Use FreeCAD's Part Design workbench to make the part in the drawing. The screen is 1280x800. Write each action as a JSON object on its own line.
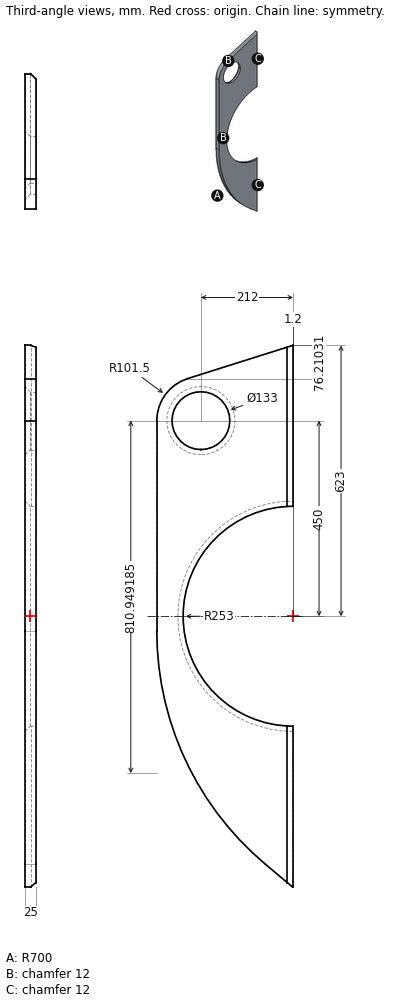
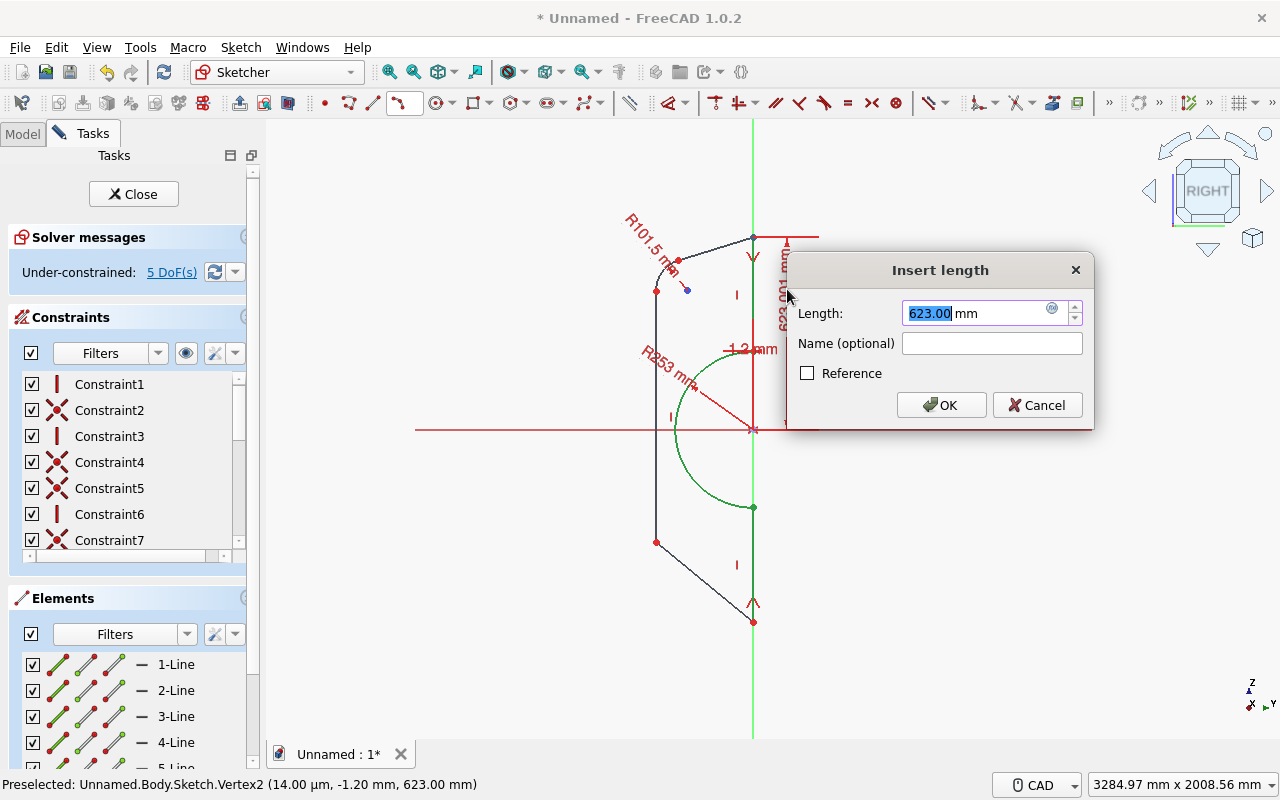
{"action": "type", "text": "623"}
{"action": "key", "text": "Return"}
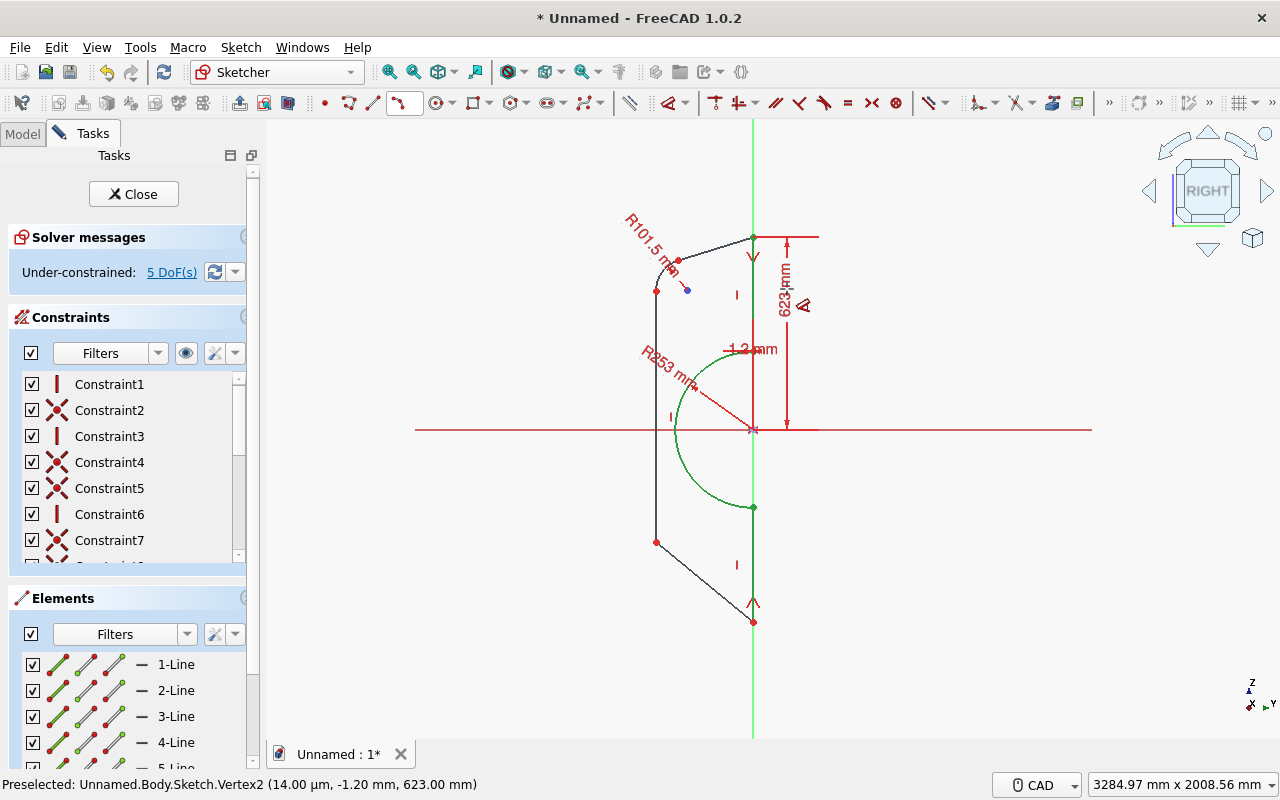
{"action": "left_click", "coordinate": [656, 292]}
{"action": "left_click", "coordinate": [622, 329]}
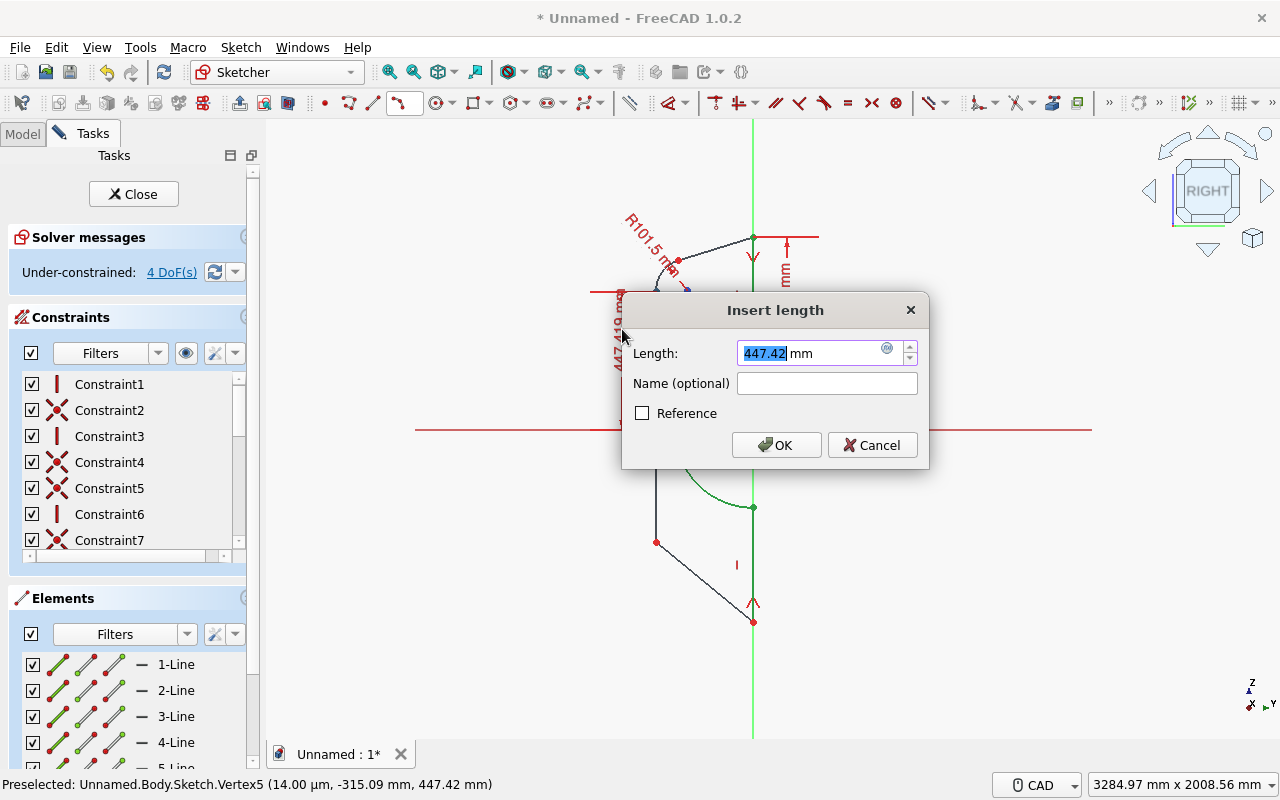
{"action": "type", "text": "450"}
{"action": "key", "text": "Return"}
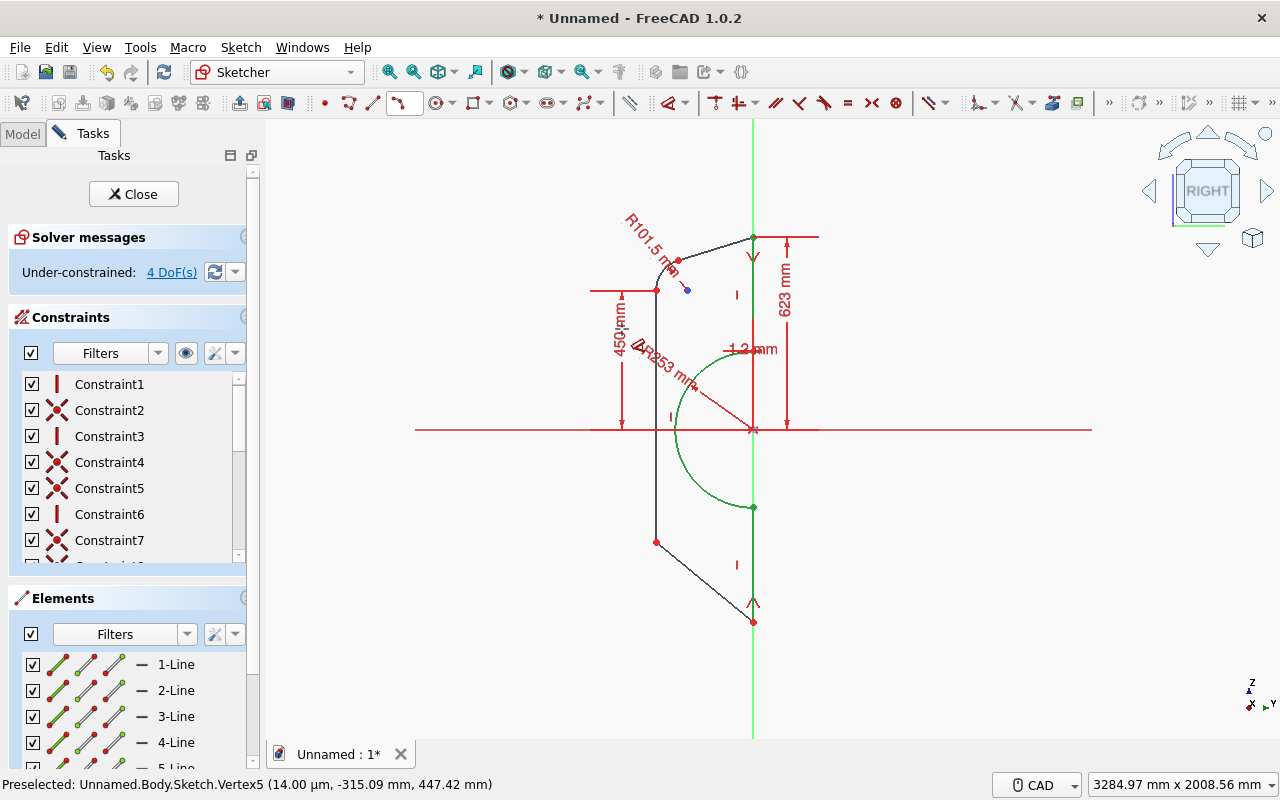
{"action": "left_click", "coordinate": [687, 290]}
{"action": "left_click", "coordinate": [736, 256]}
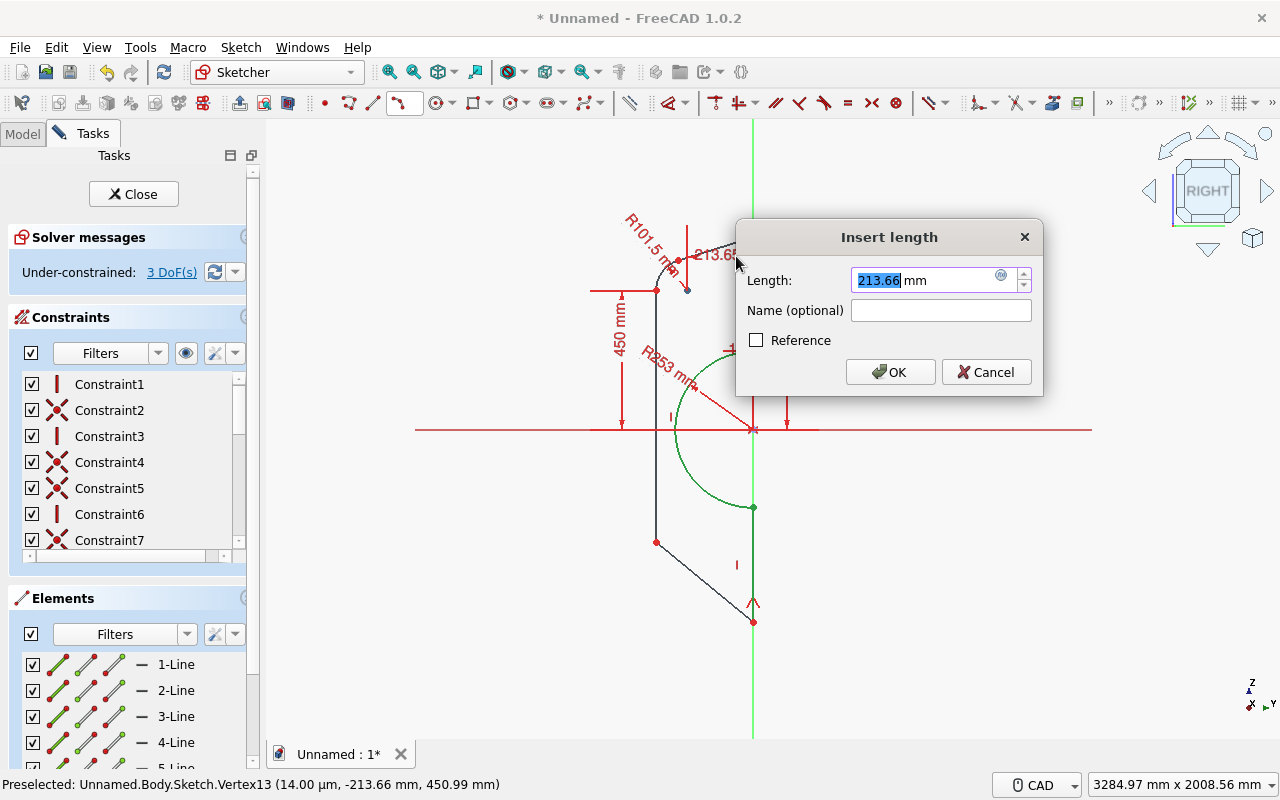
{"action": "type", "text": "212"}
{"action": "key", "text": "Return"}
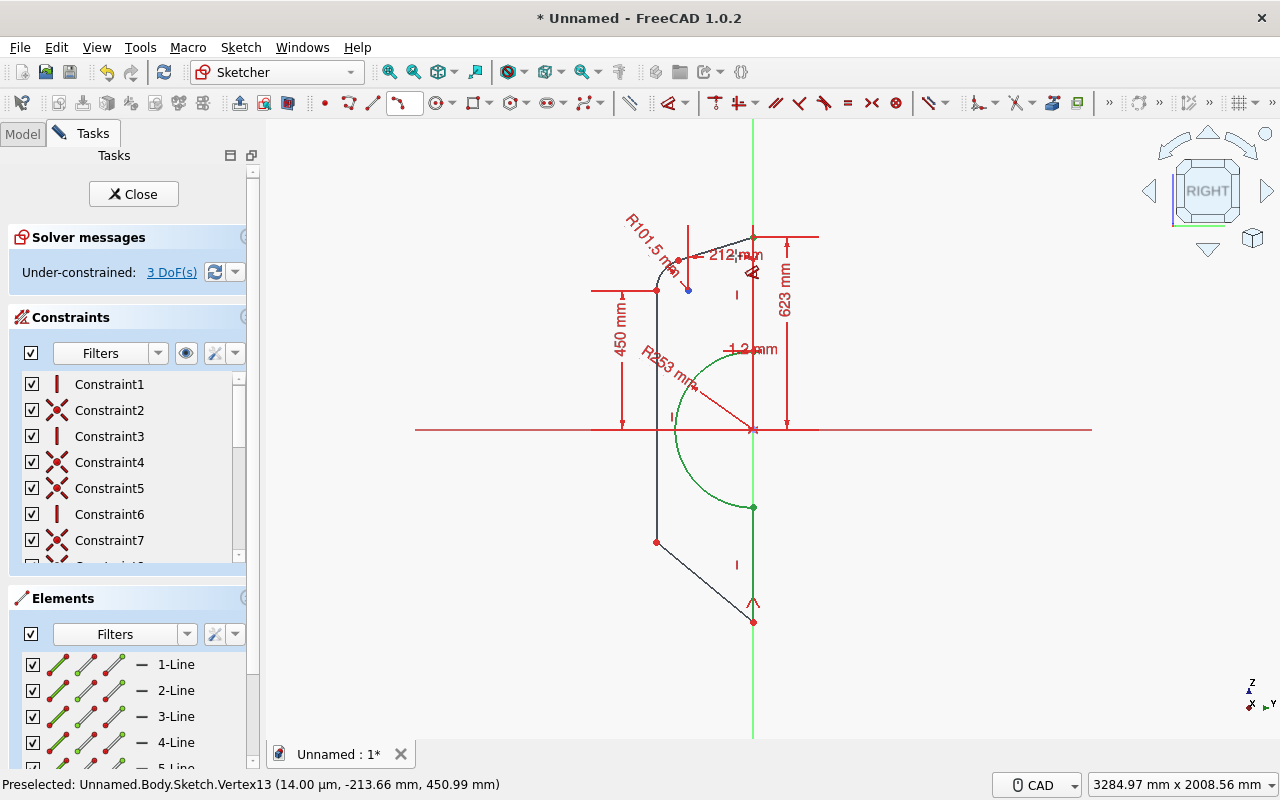
{"action": "left_click", "coordinate": [688, 290]}
{"action": "left_click", "coordinate": [787, 328]}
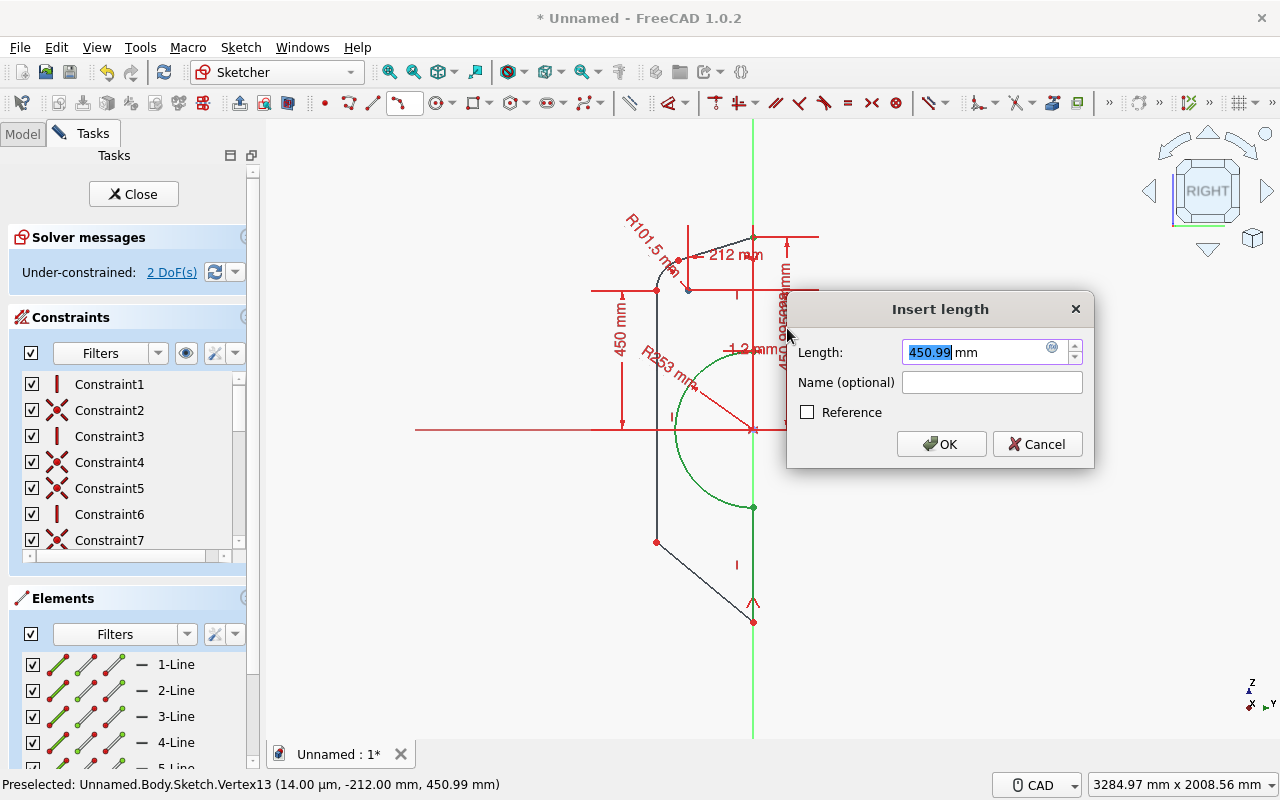
{"action": "type", "text": "450"}
{"action": "key", "text": "Return"}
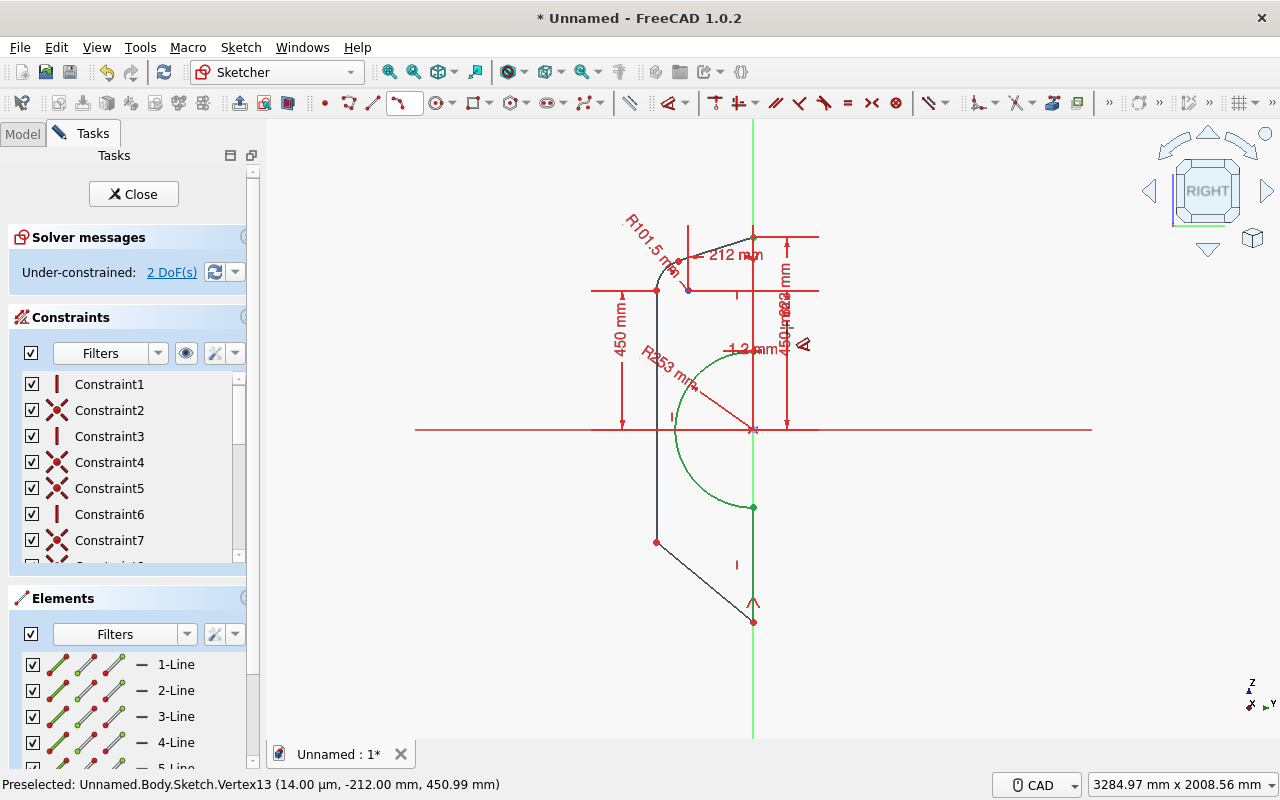
{"action": "scroll", "coordinate": [731, 244], "scroll_direction": "up", "scroll_amount": 3}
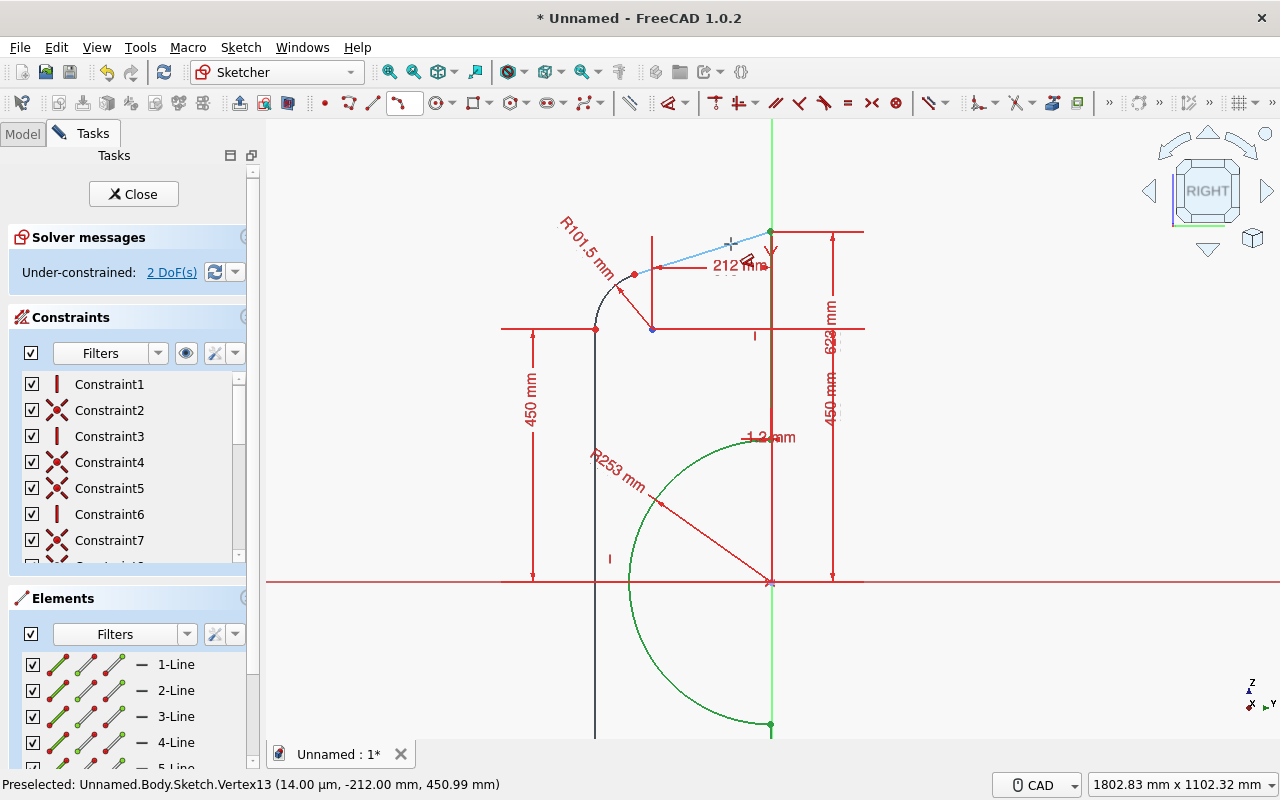
{"action": "left_click", "coordinate": [730, 245]}
{"action": "left_click", "coordinate": [805, 243]}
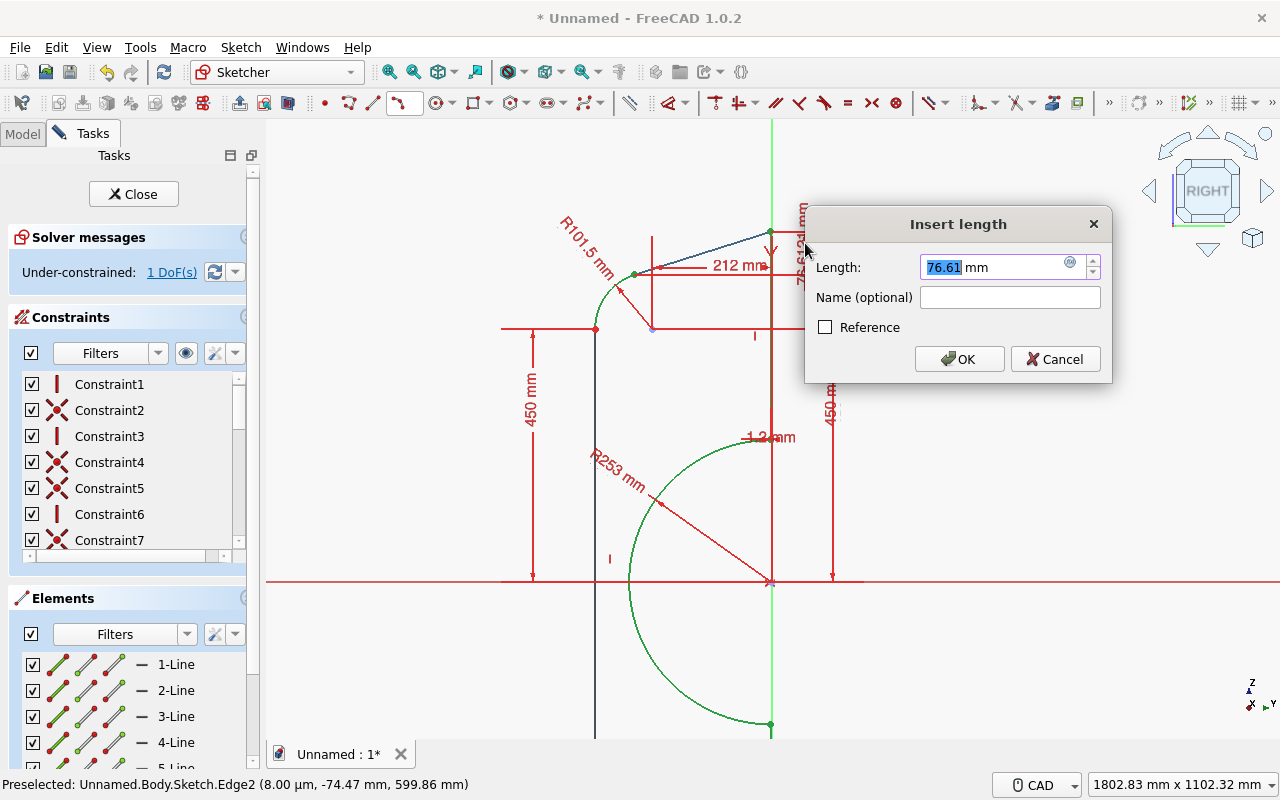
{"action": "type", "text": "76.21031"}
{"action": "key", "text": "Return"}